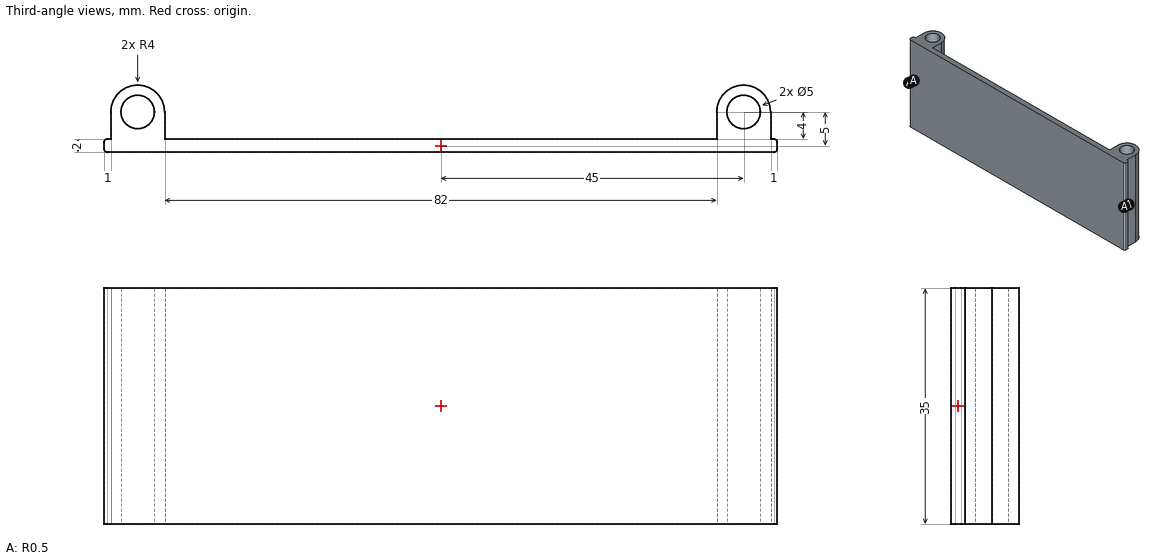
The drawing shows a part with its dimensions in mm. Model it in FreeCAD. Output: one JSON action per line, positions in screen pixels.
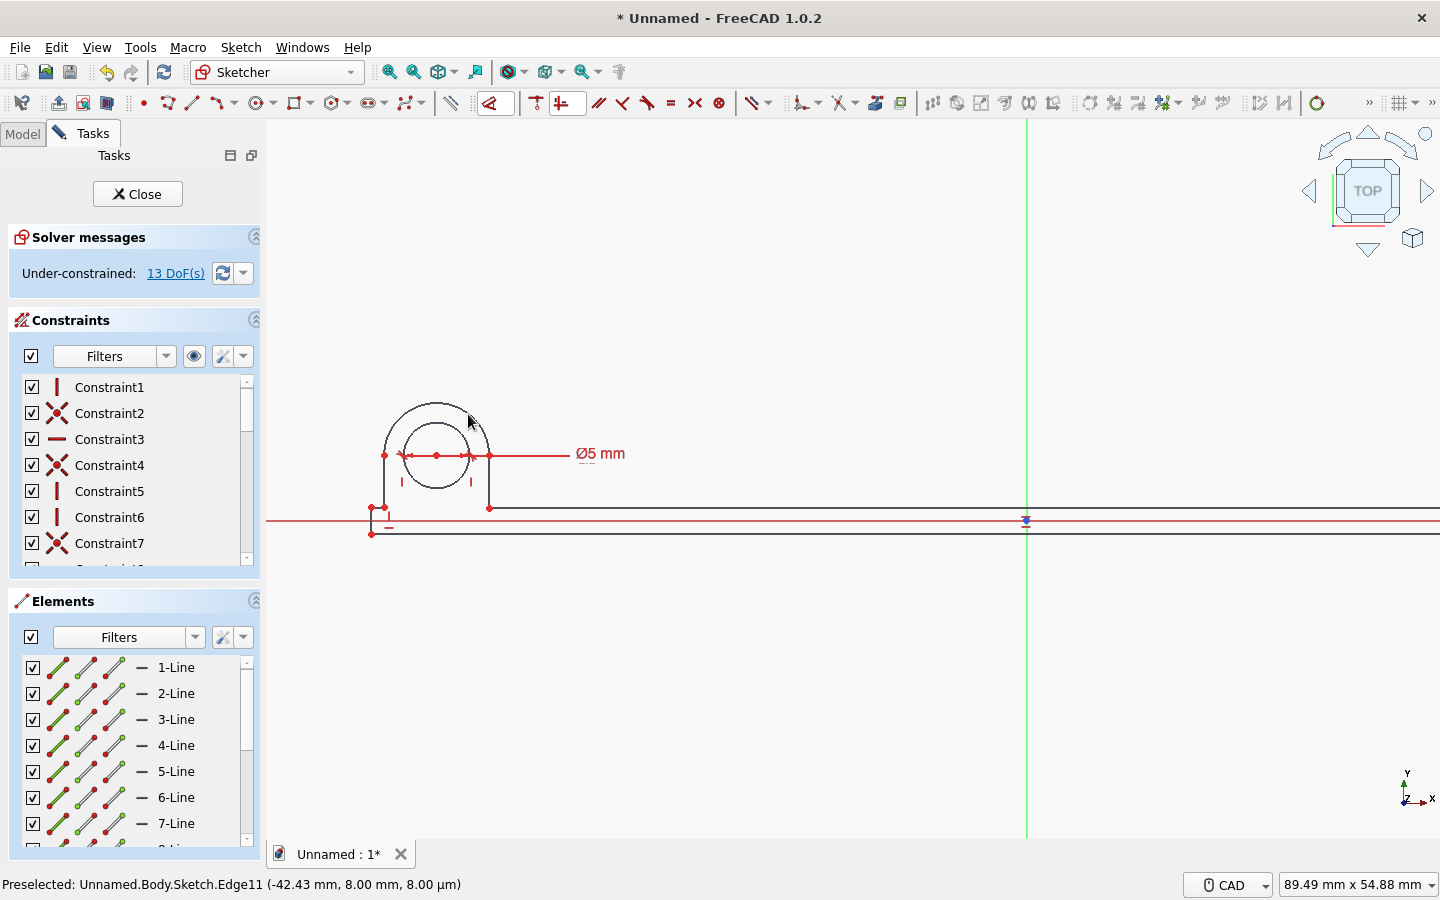
{"action": "scroll", "coordinate": [490, 492], "scroll_direction": "down", "scroll_amount": 3}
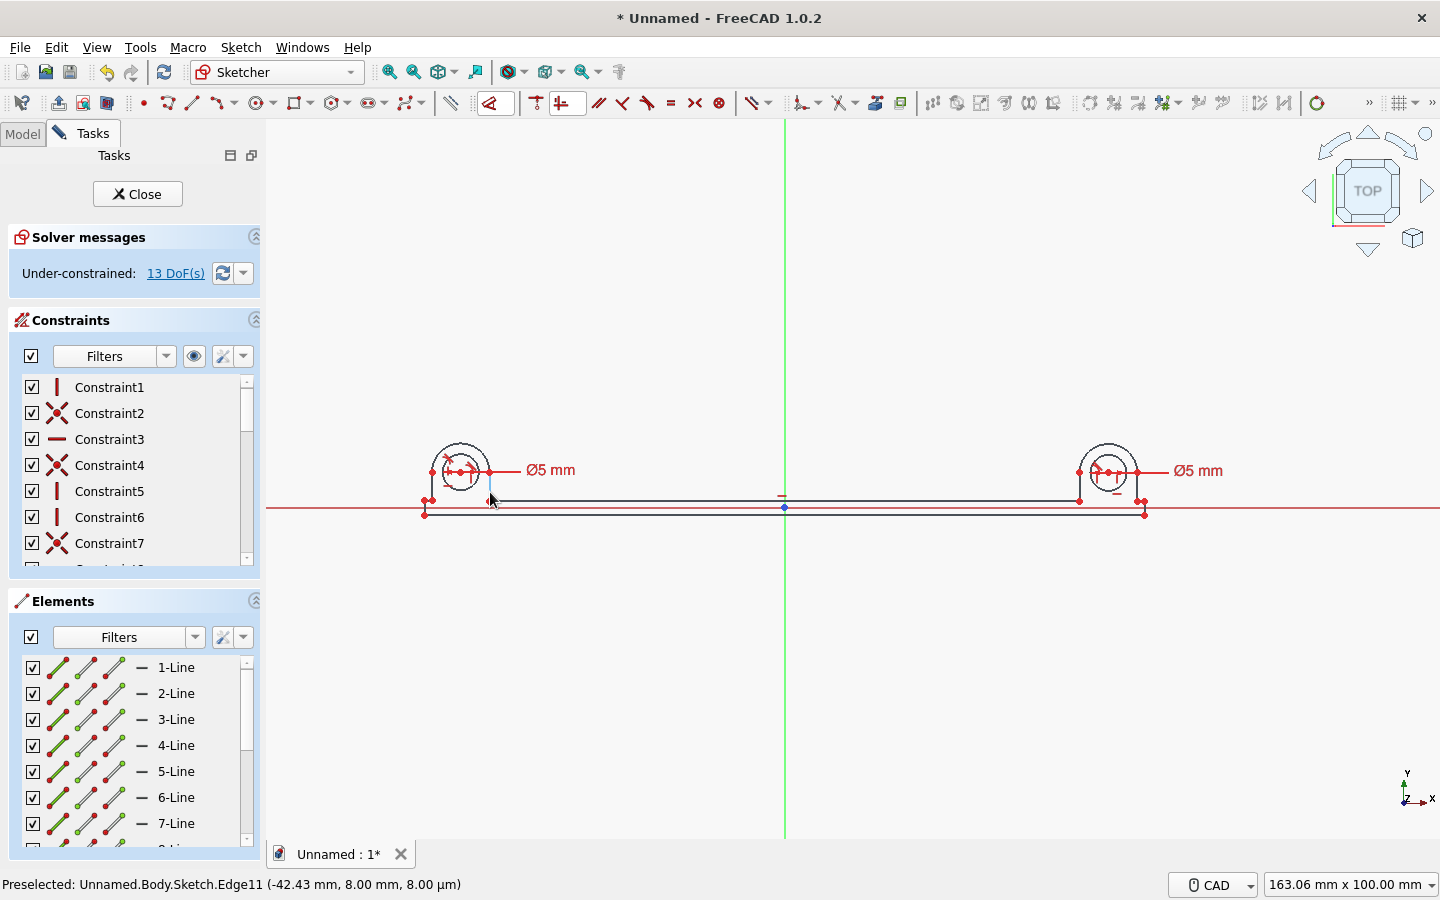
{"action": "scroll", "coordinate": [1137, 492], "scroll_direction": "up", "scroll_amount": 3}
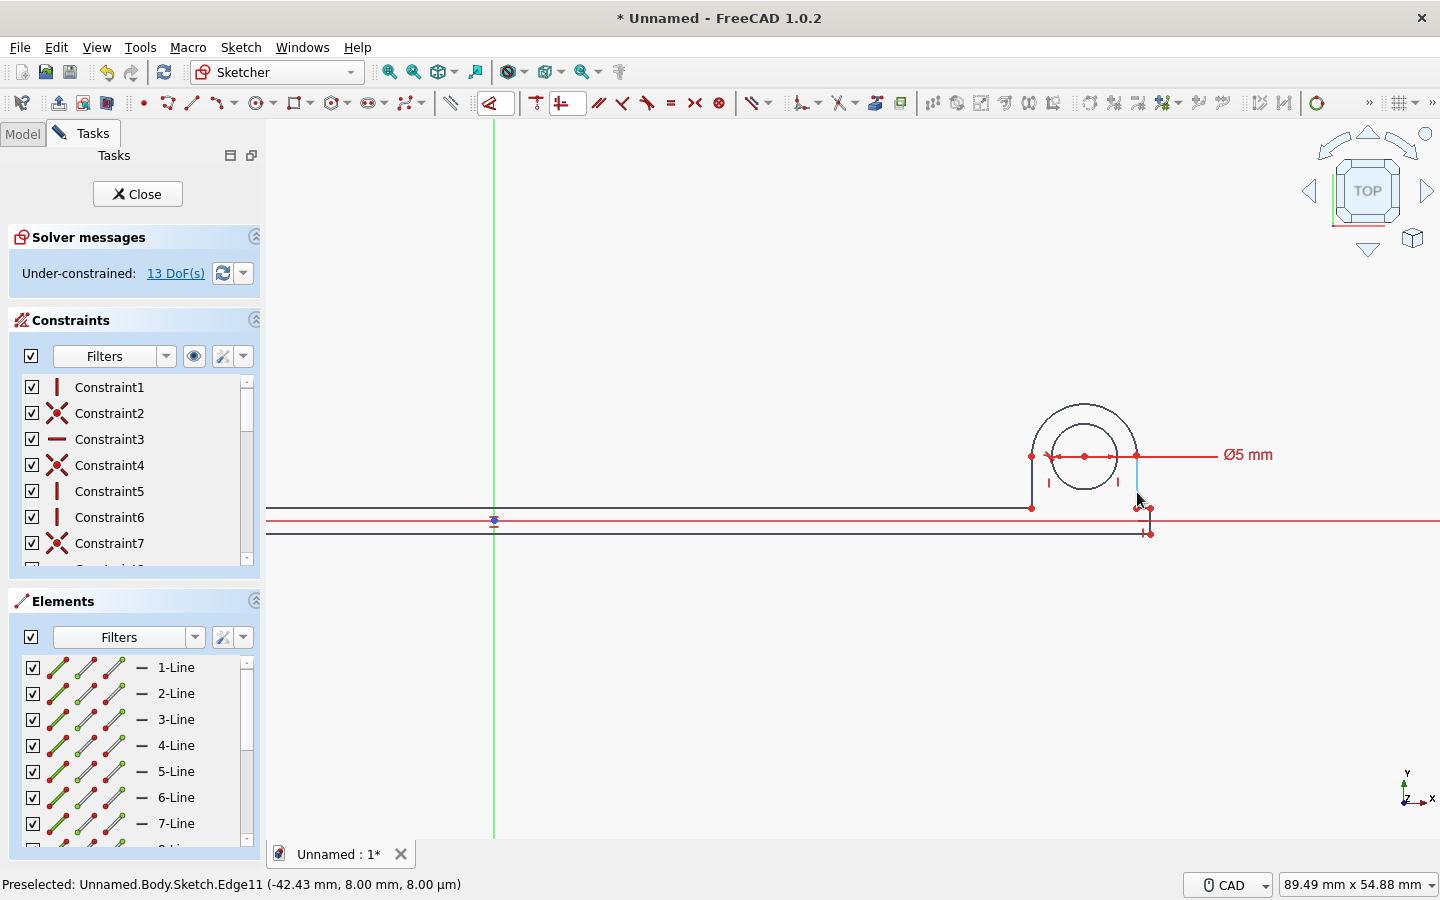
{"action": "left_click", "coordinate": [1137, 492]}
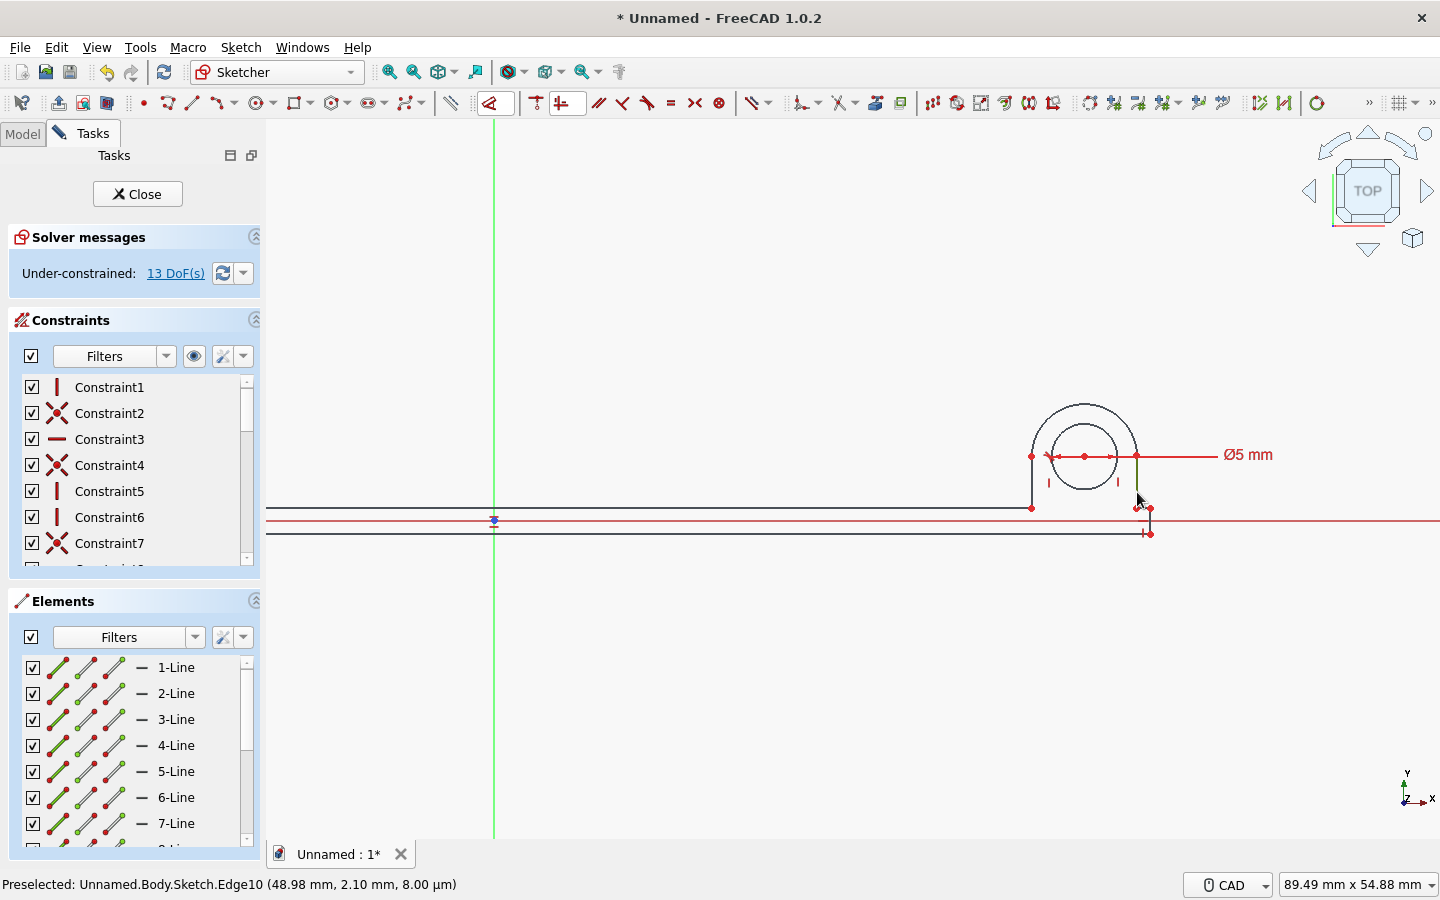
{"action": "left_click", "coordinate": [1115, 414]}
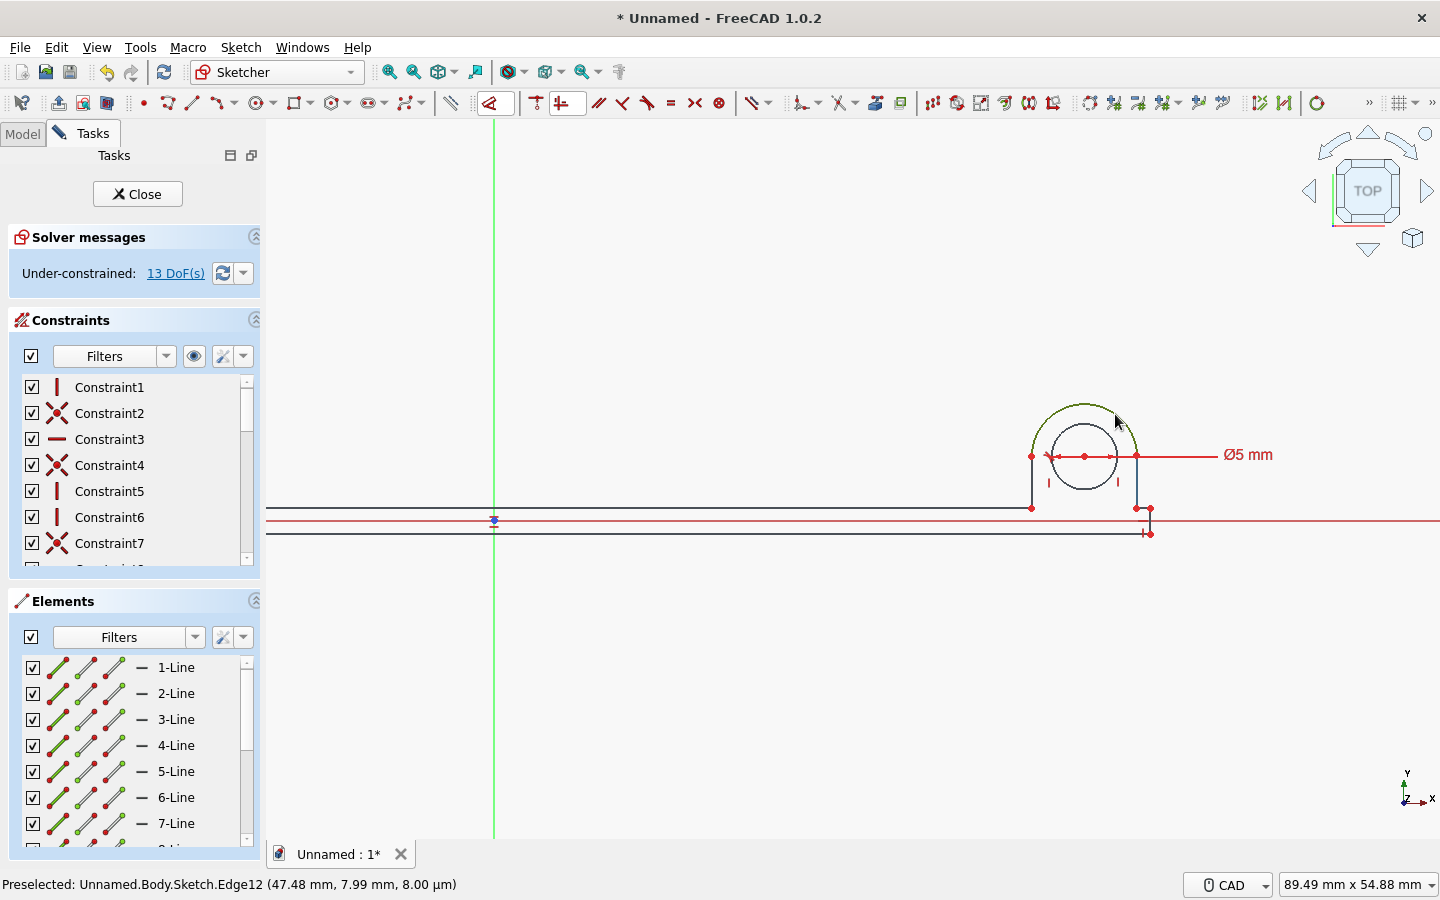
{"action": "left_click", "coordinate": [648, 104]}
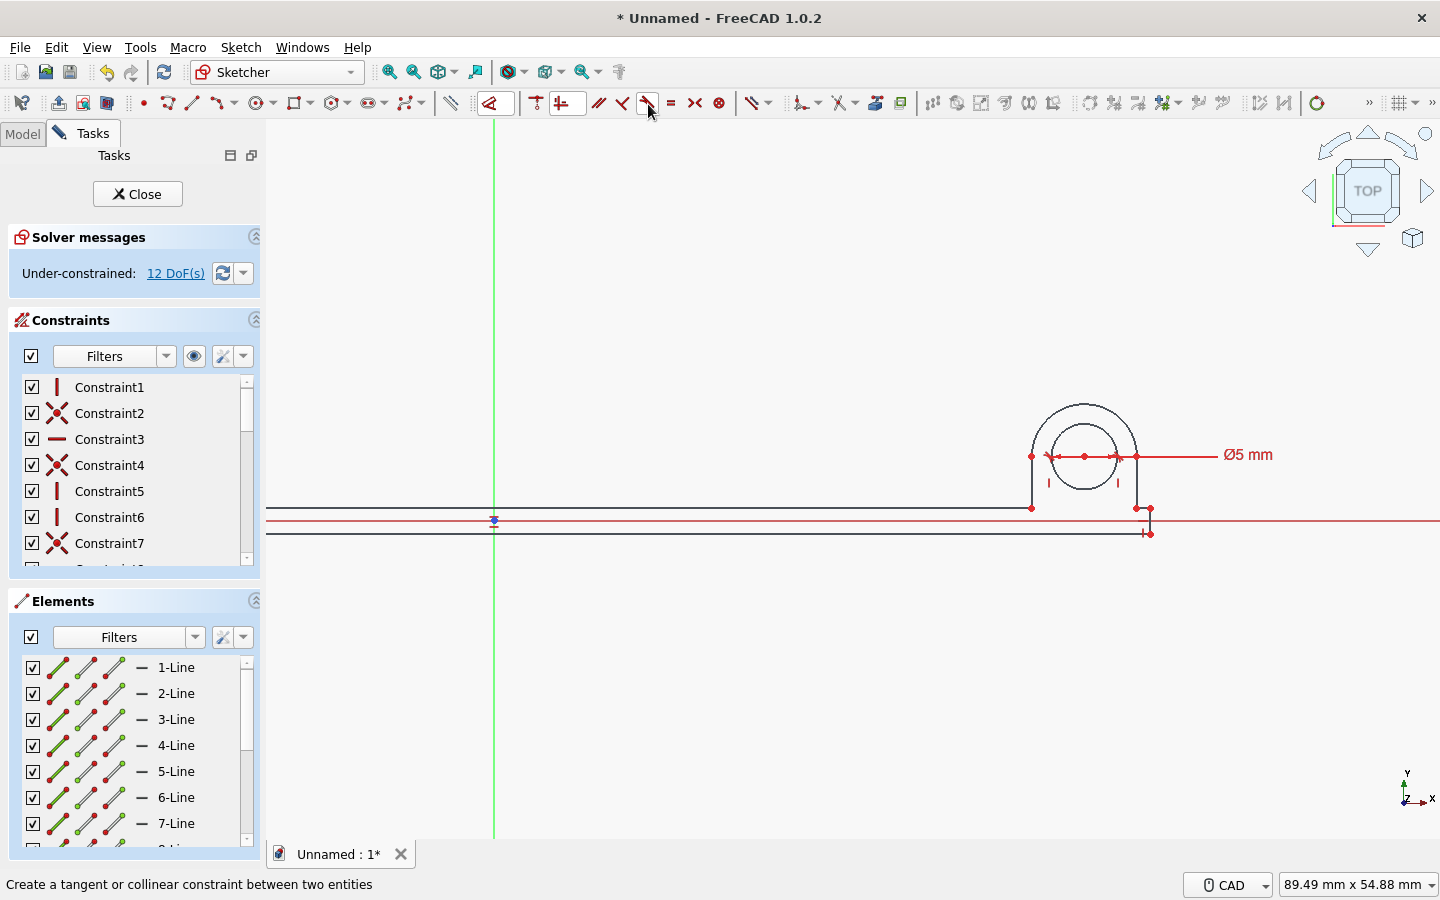
{"action": "scroll", "coordinate": [1137, 492], "scroll_direction": "down", "scroll_amount": 3}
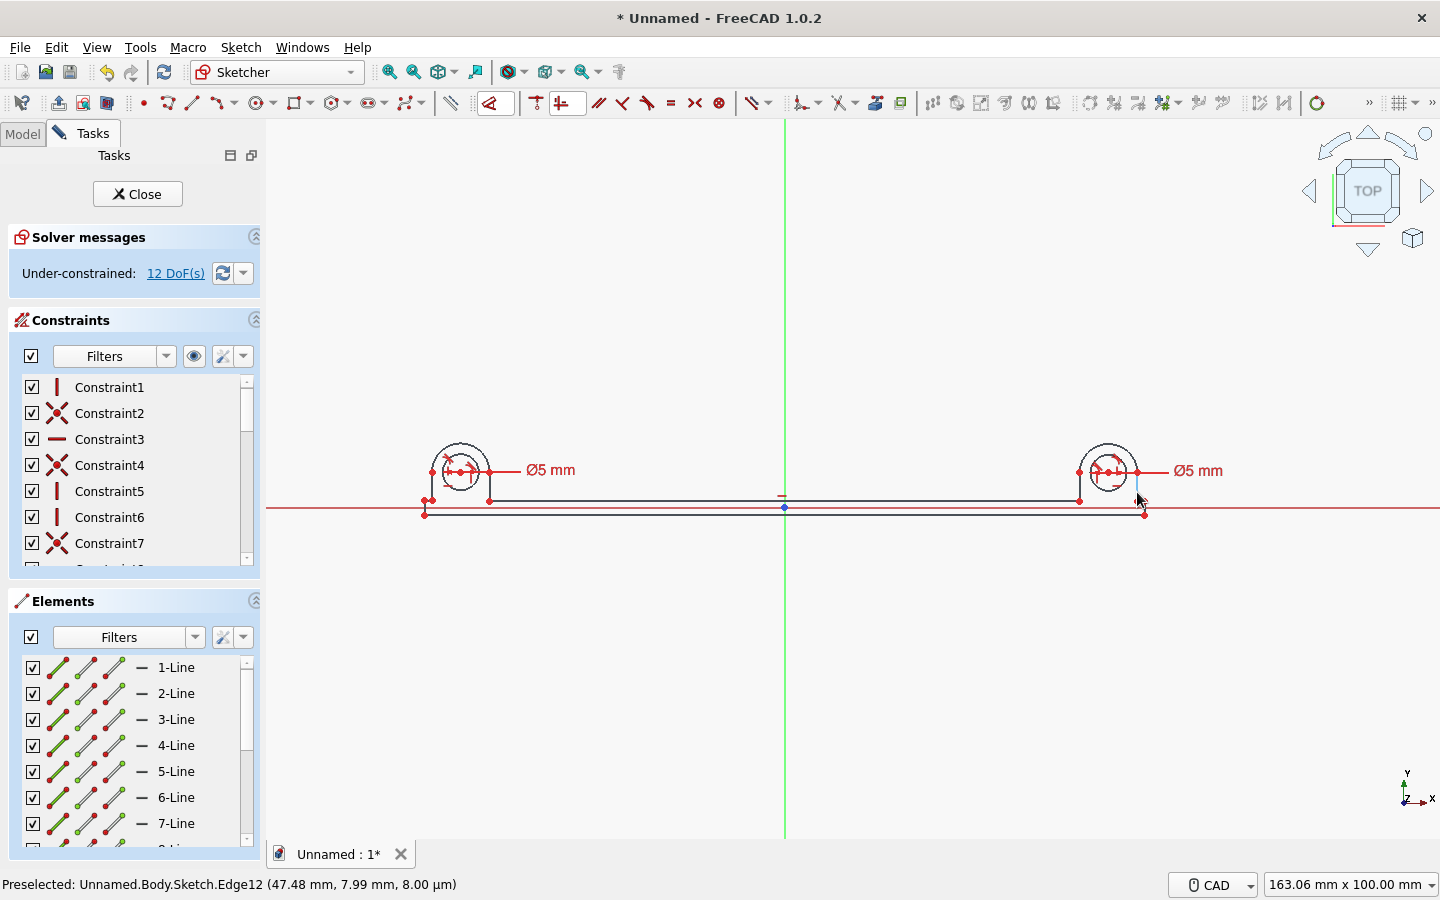
{"action": "scroll", "coordinate": [478, 449], "scroll_direction": "up", "scroll_amount": 2}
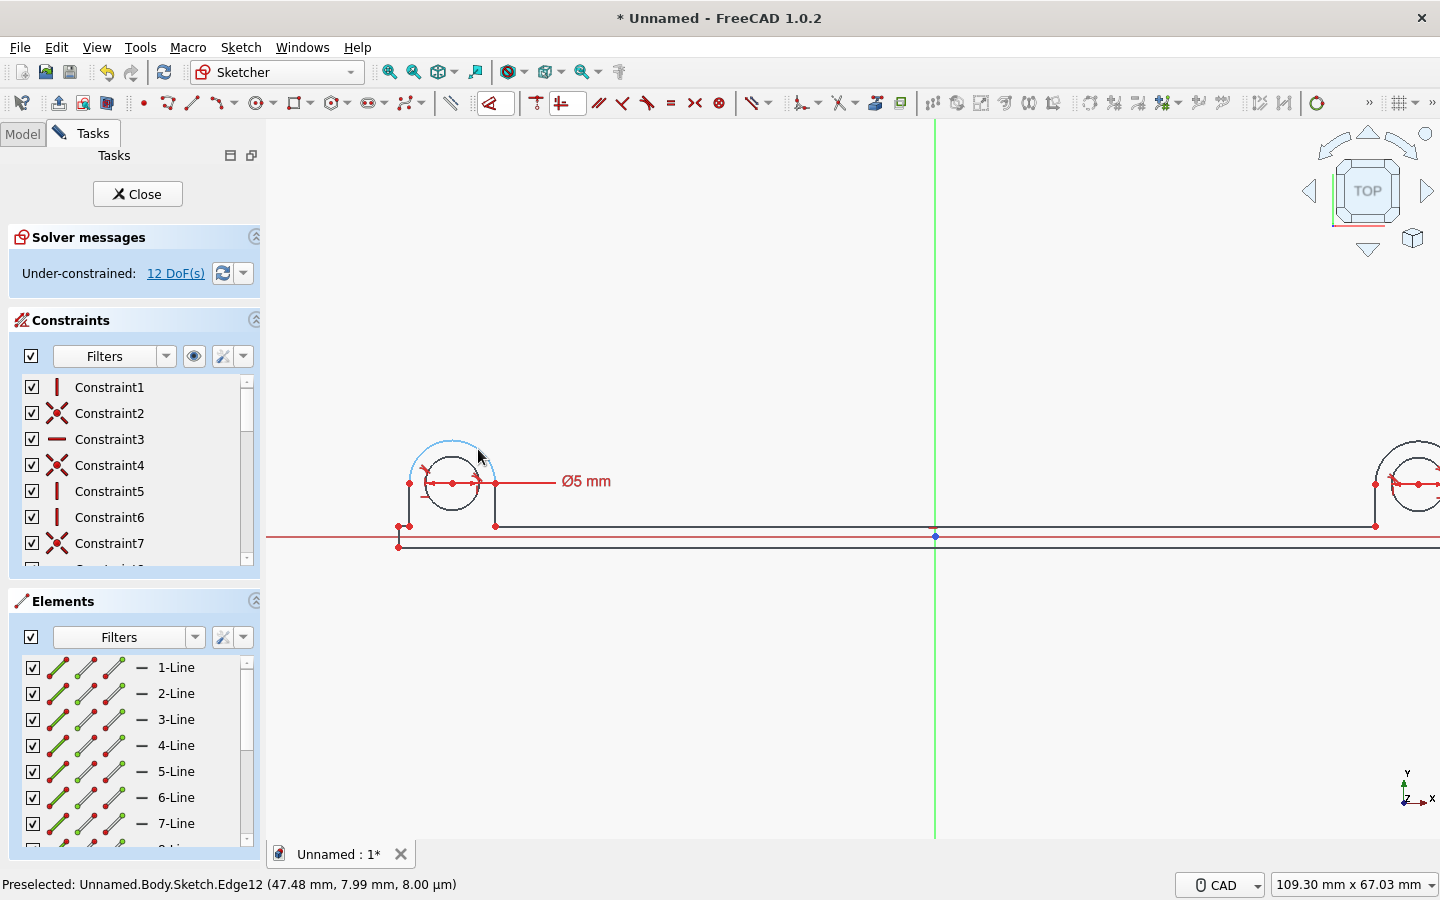
{"action": "left_click", "coordinate": [477, 449]}